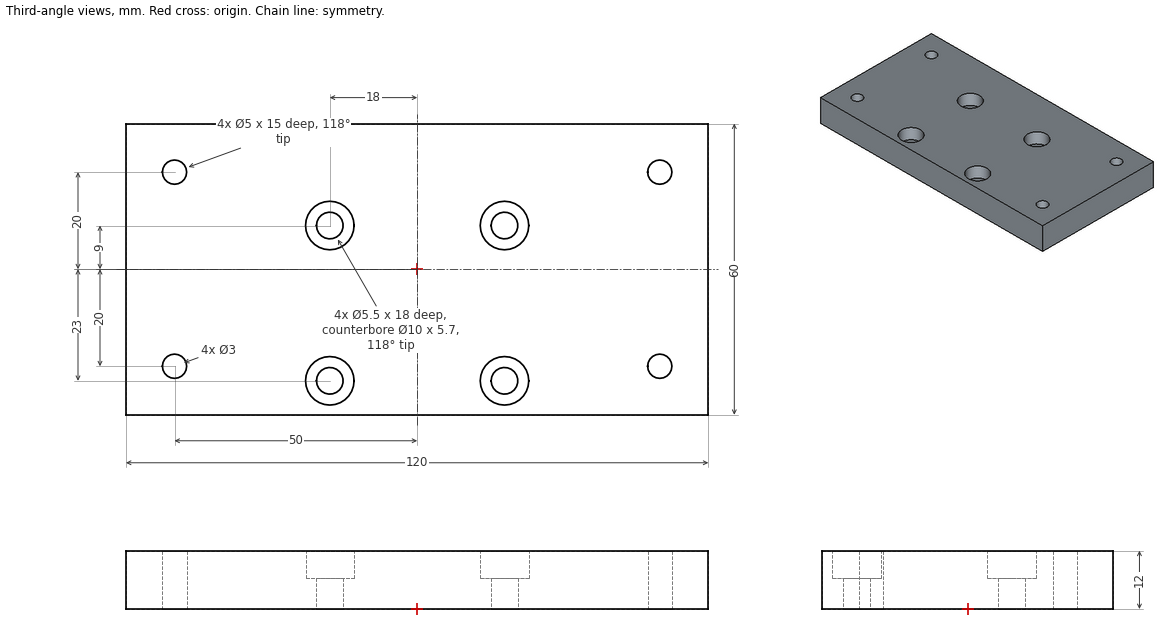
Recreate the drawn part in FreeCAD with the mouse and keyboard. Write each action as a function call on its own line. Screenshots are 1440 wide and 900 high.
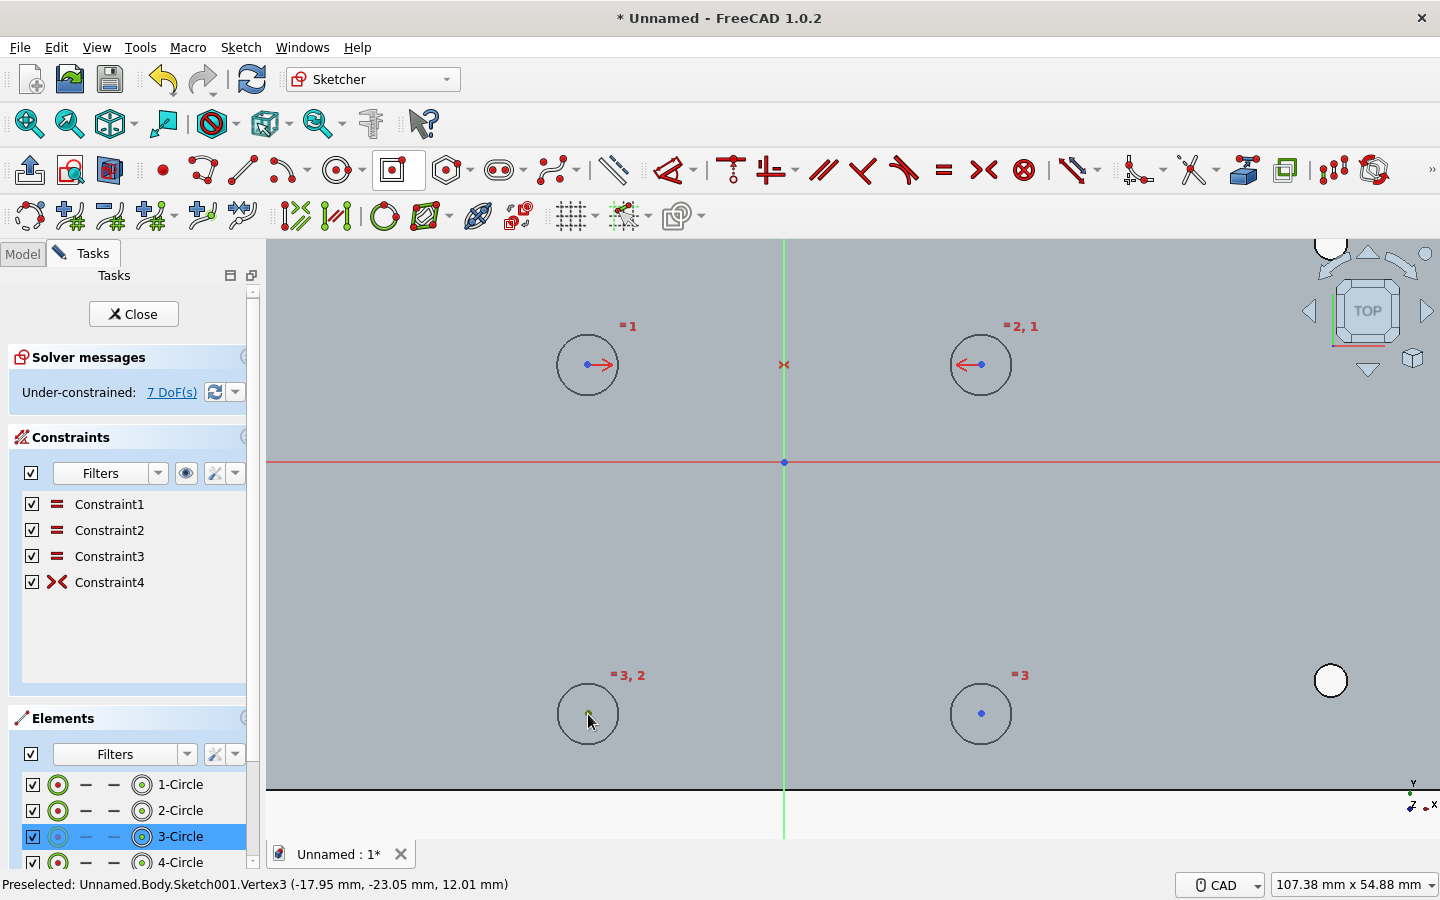
click(981, 714)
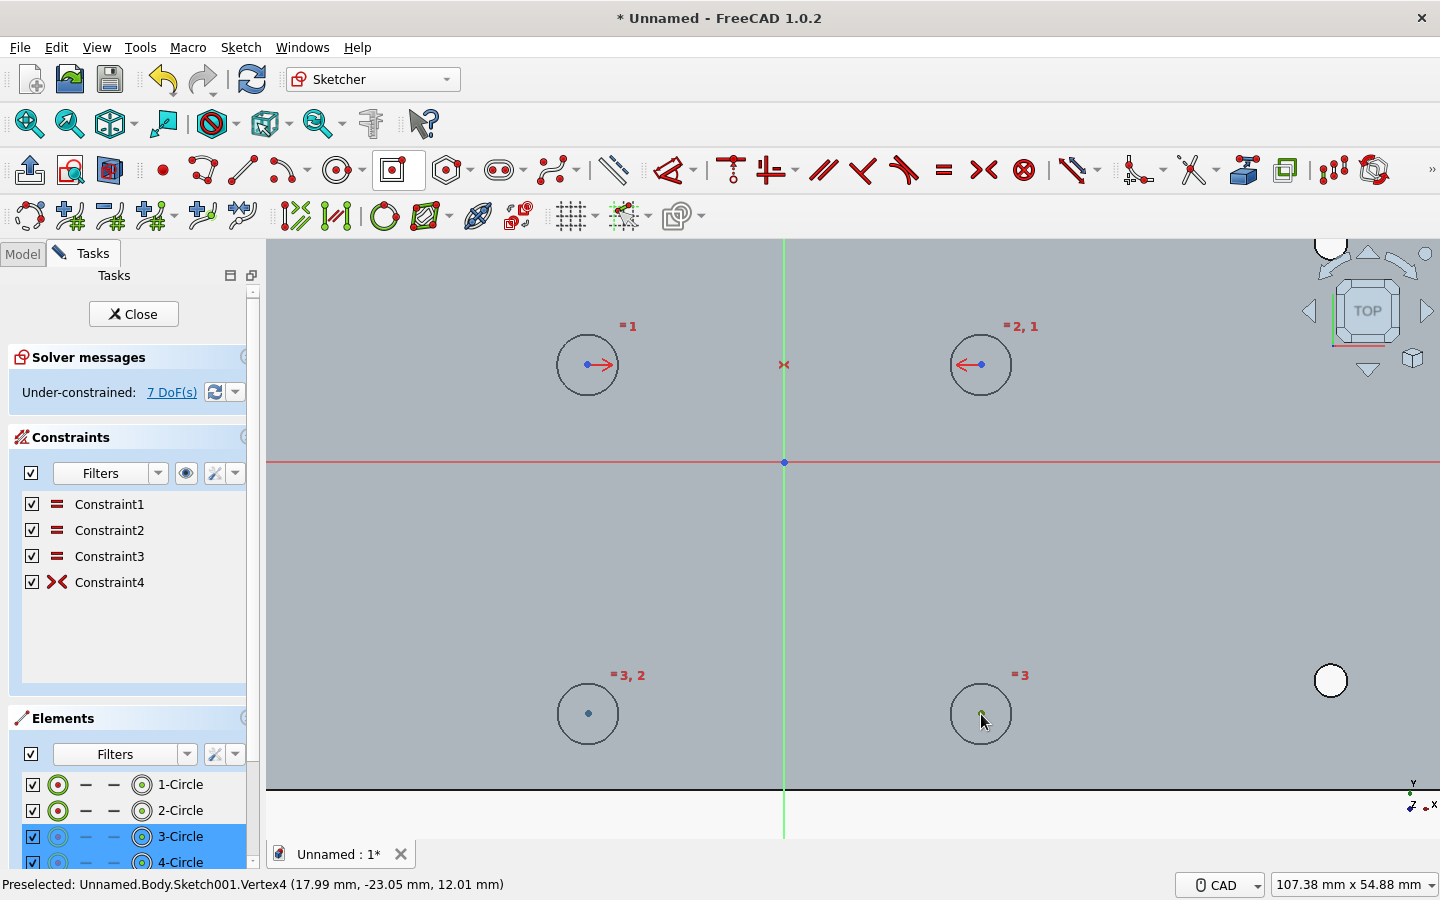
click(784, 772)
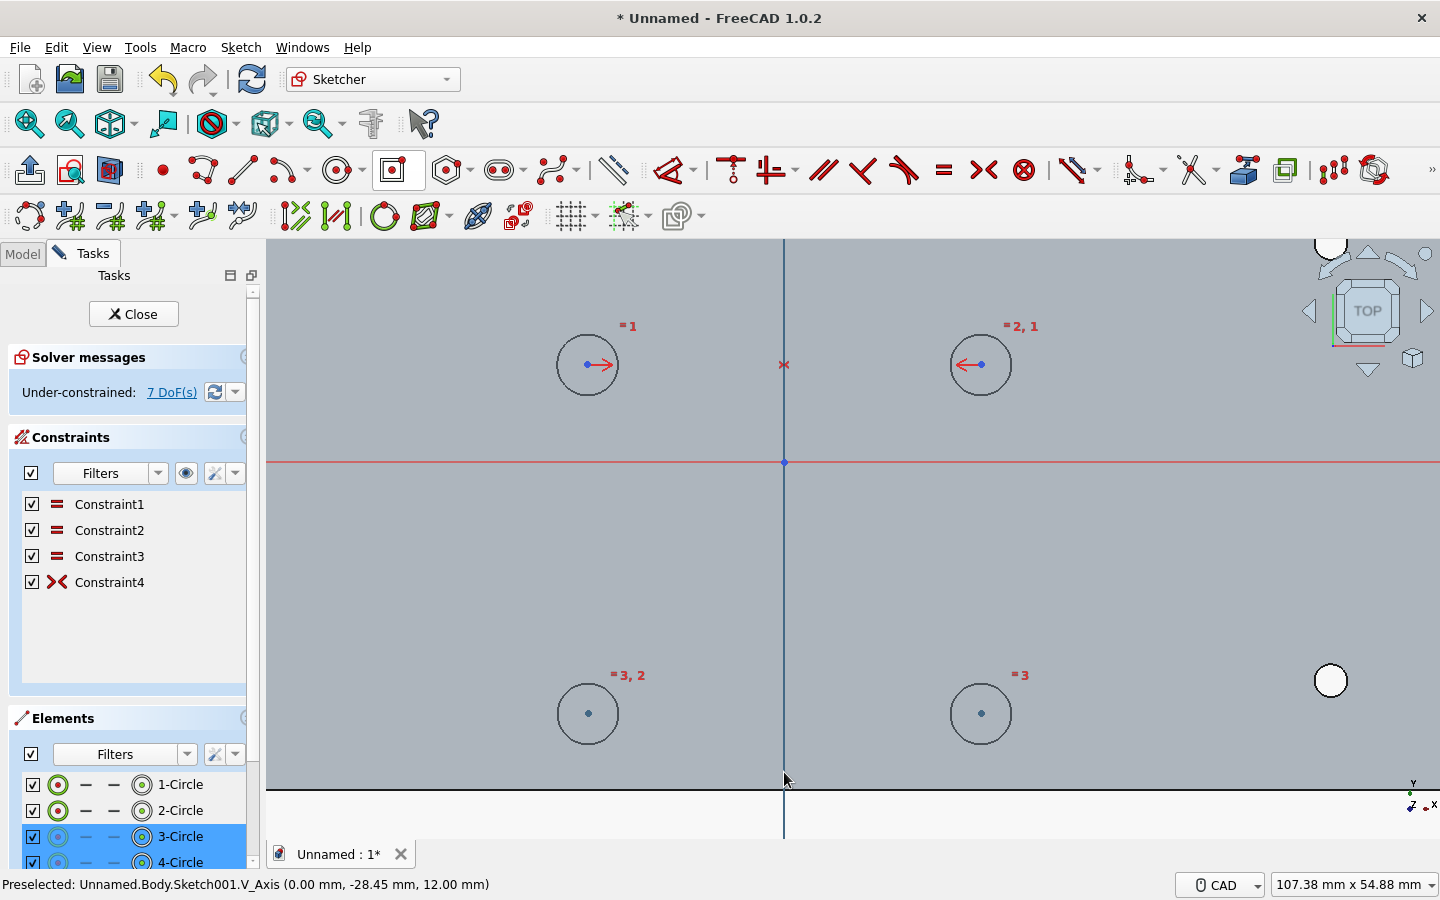
click(984, 170)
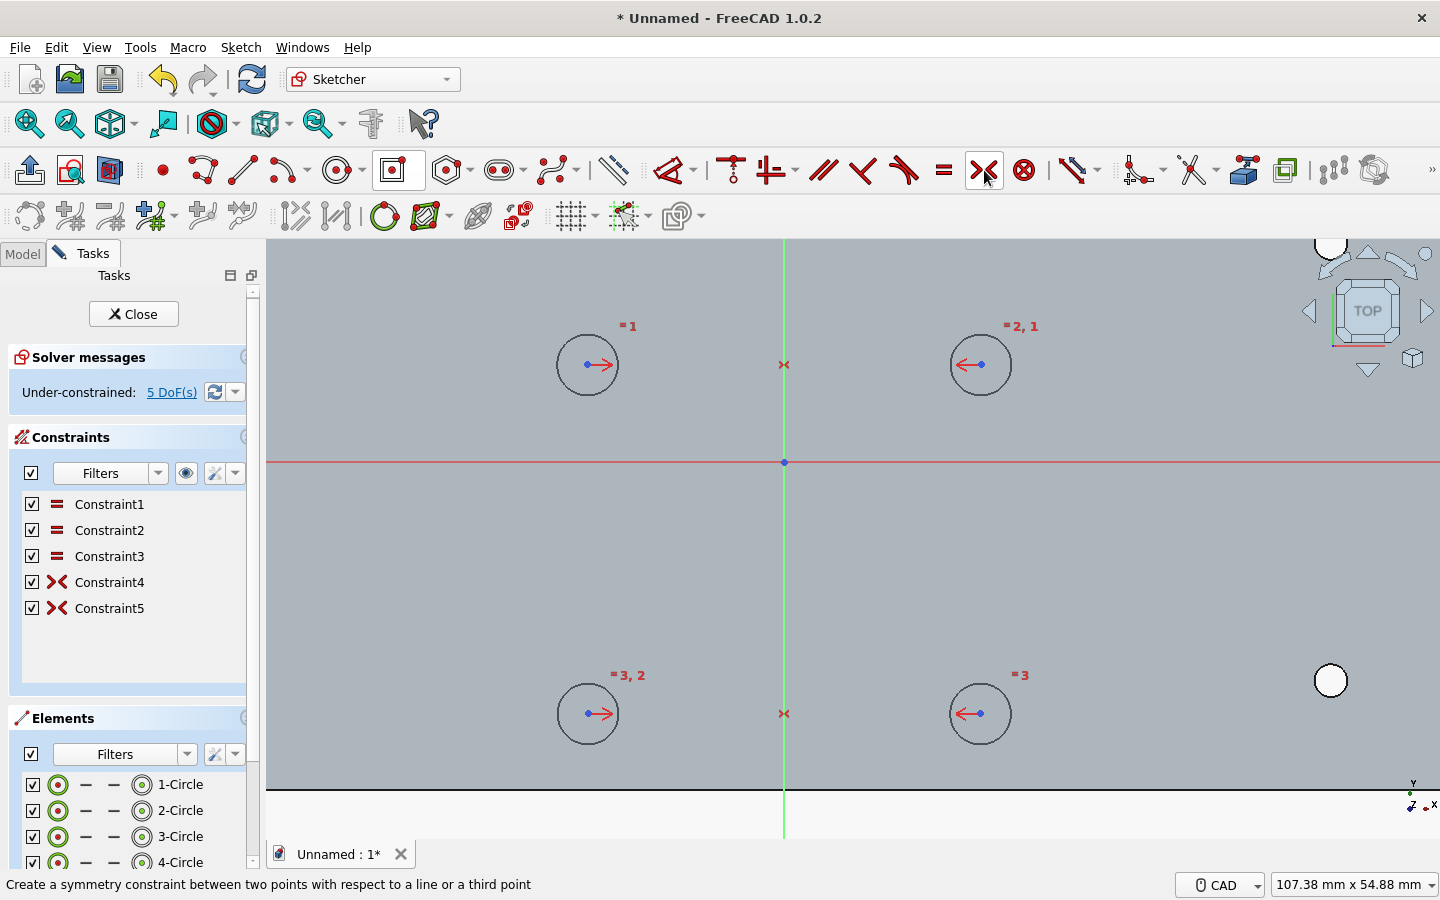
click(668, 170)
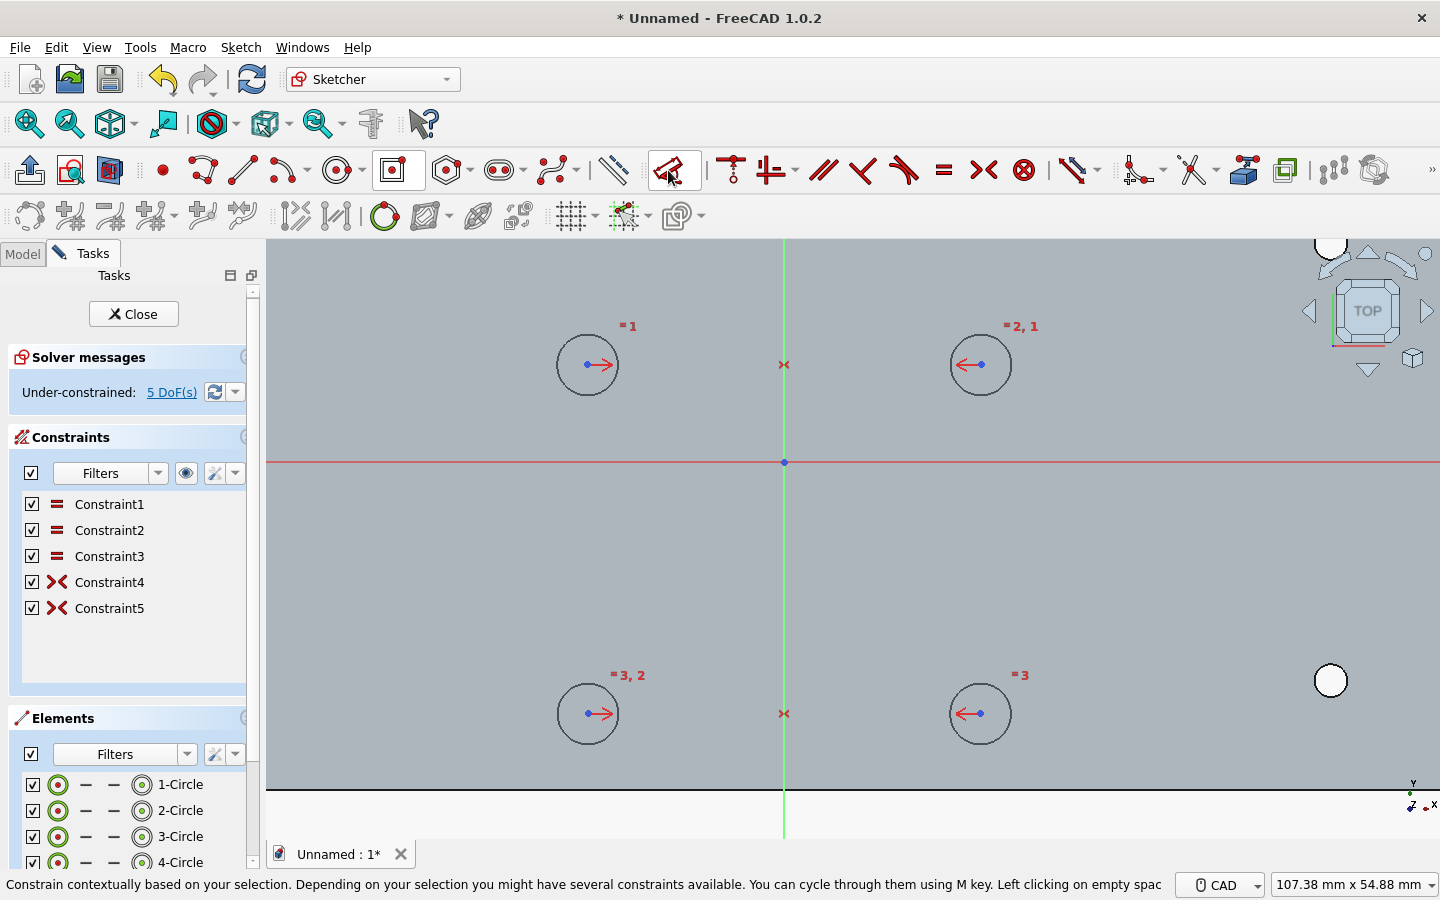
click(609, 343)
click(631, 320)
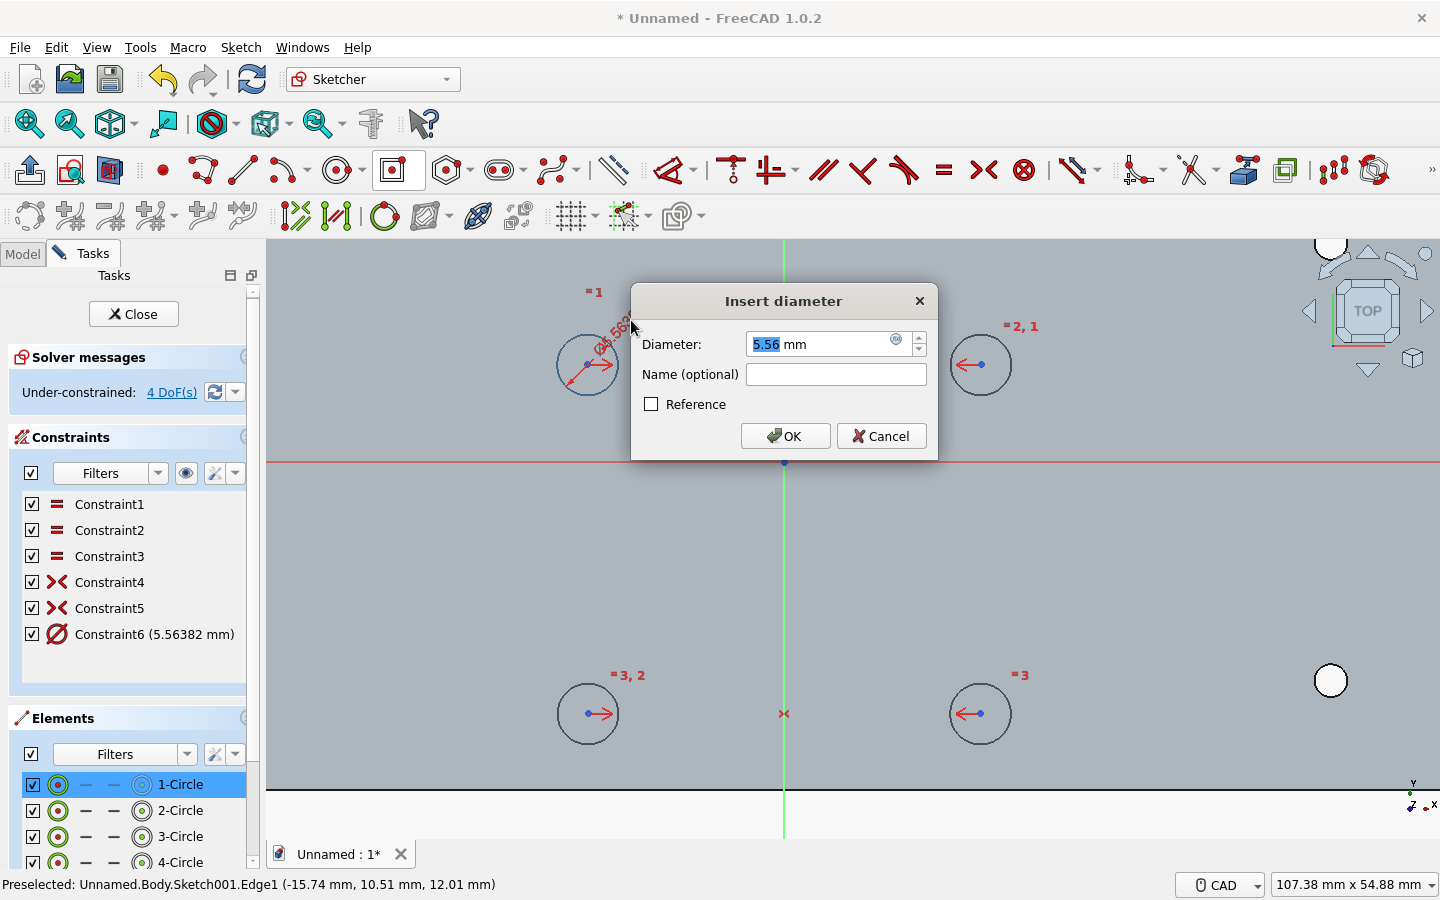
text(5.5)
key(Return)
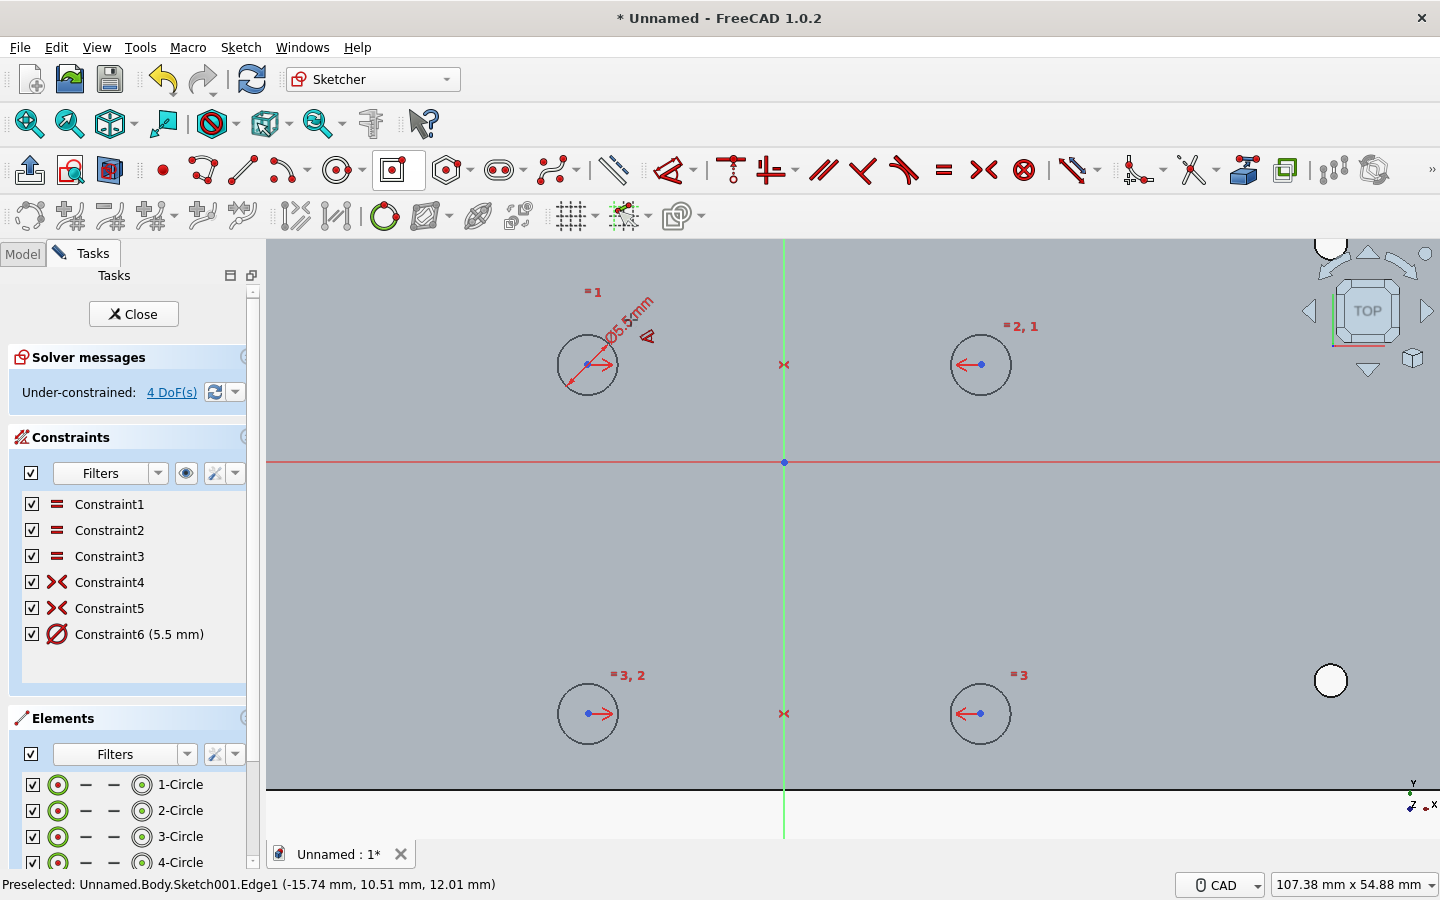
click(588, 365)
click(554, 414)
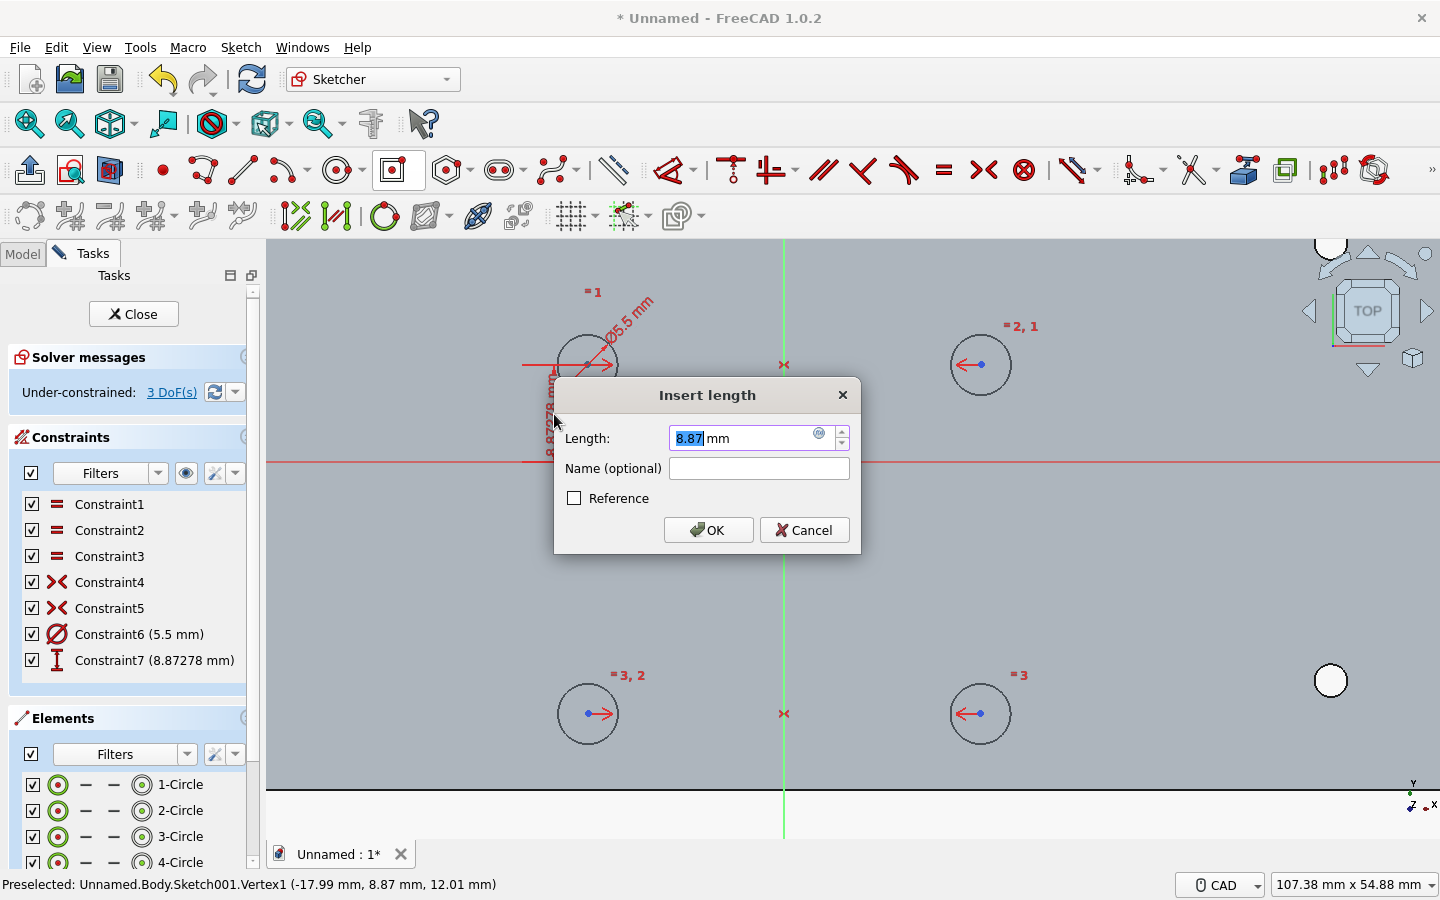
text(9)
key(Return)